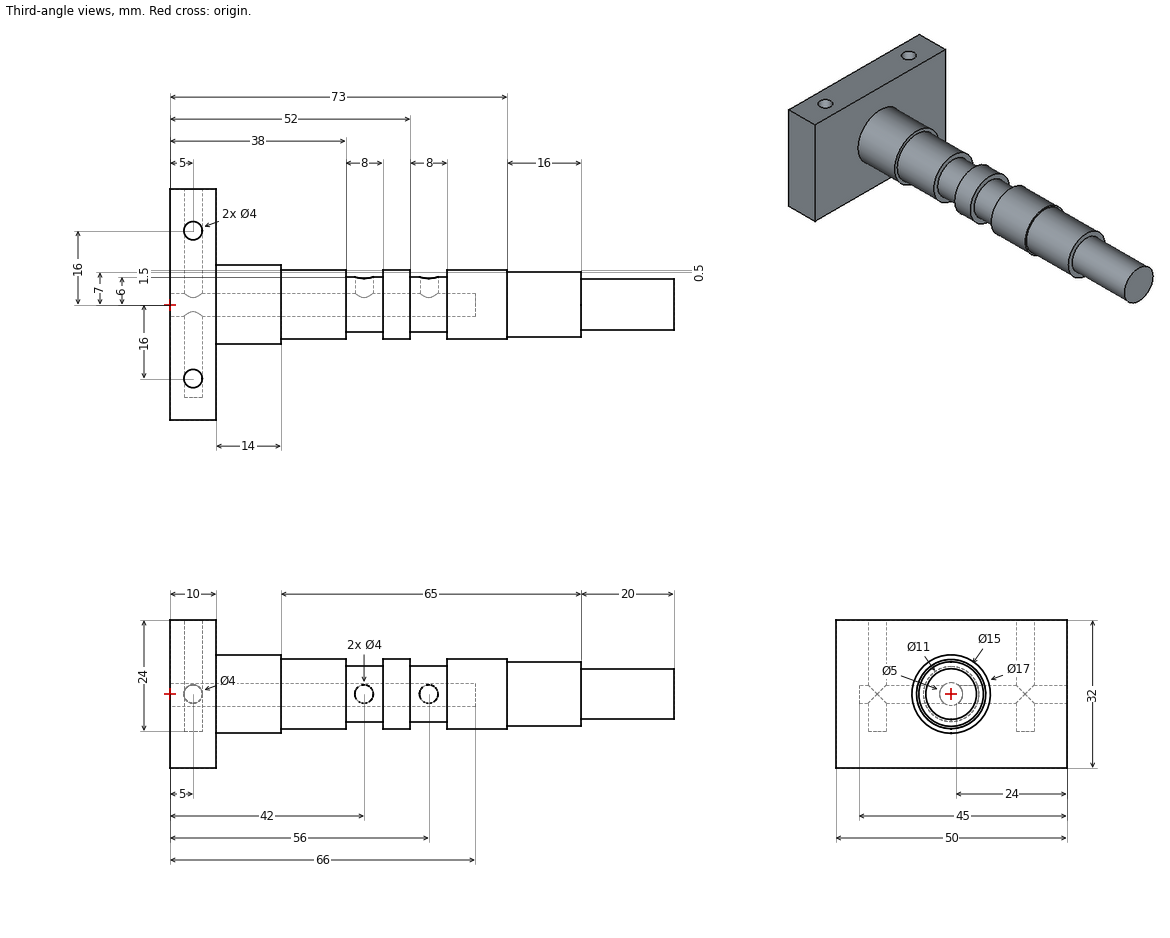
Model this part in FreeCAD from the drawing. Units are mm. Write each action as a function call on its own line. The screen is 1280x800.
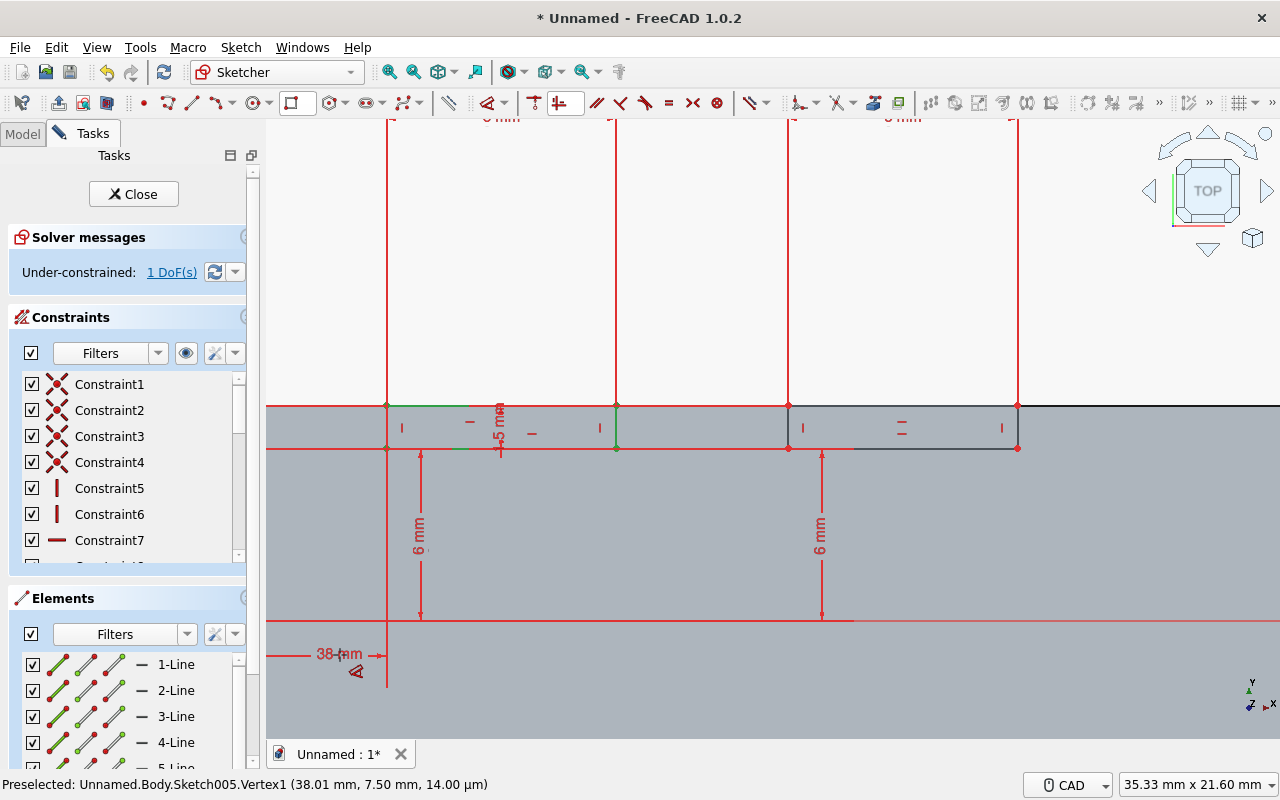
click(788, 406)
click(541, 655)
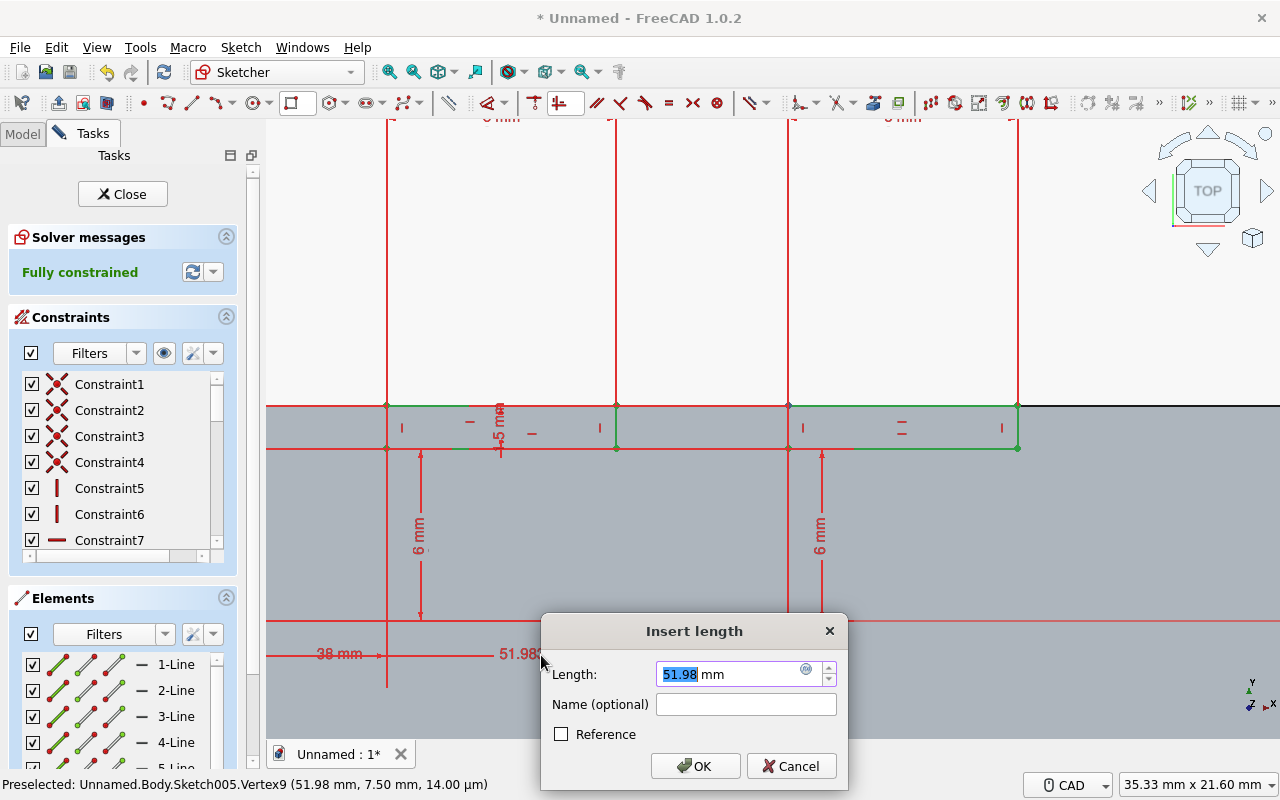
text(52)
key(Return)
key(Escape)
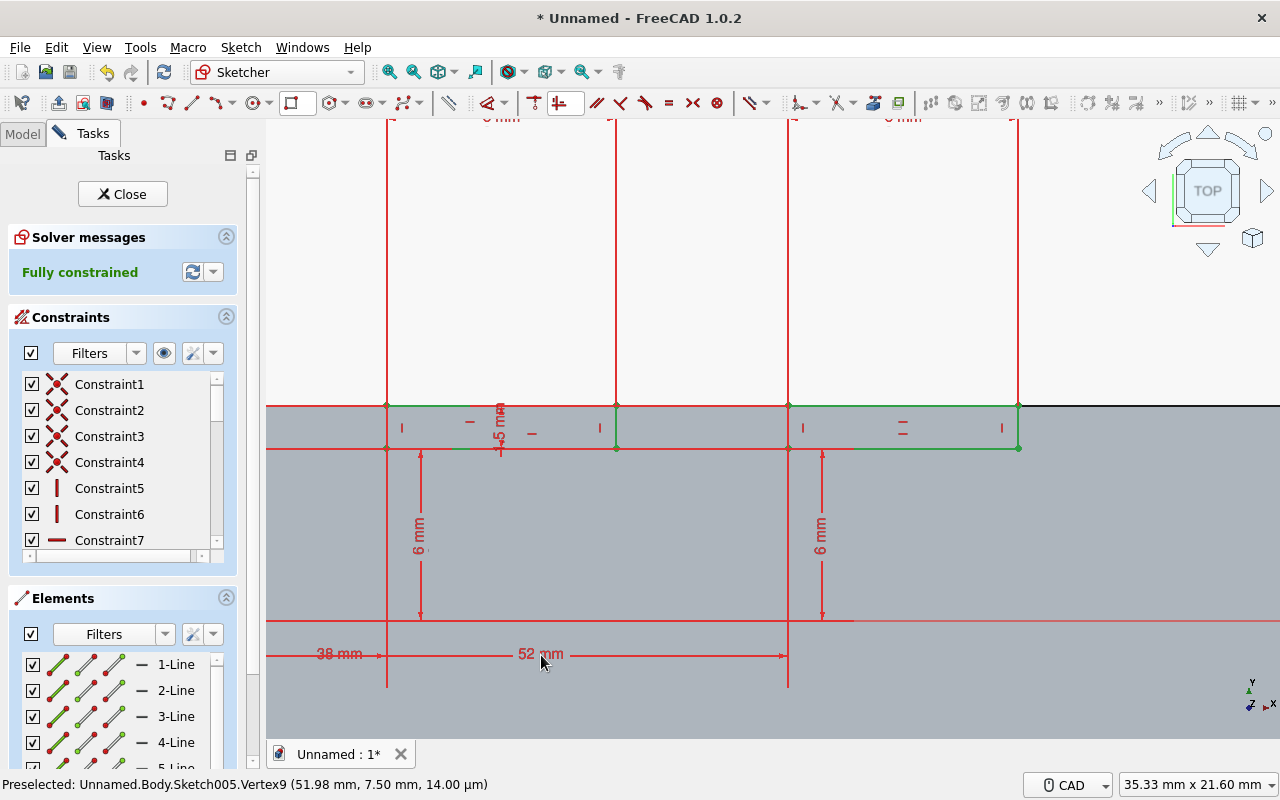
click(123, 194)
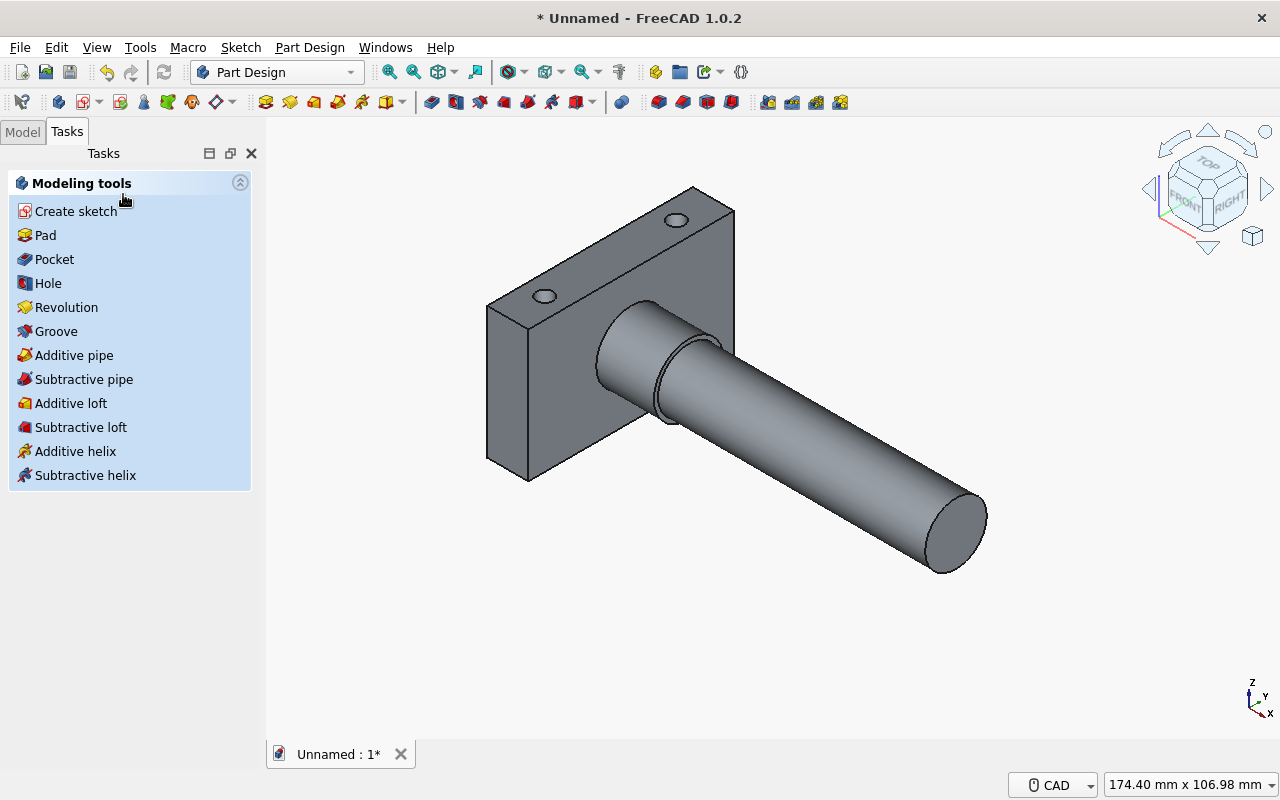
click(480, 102)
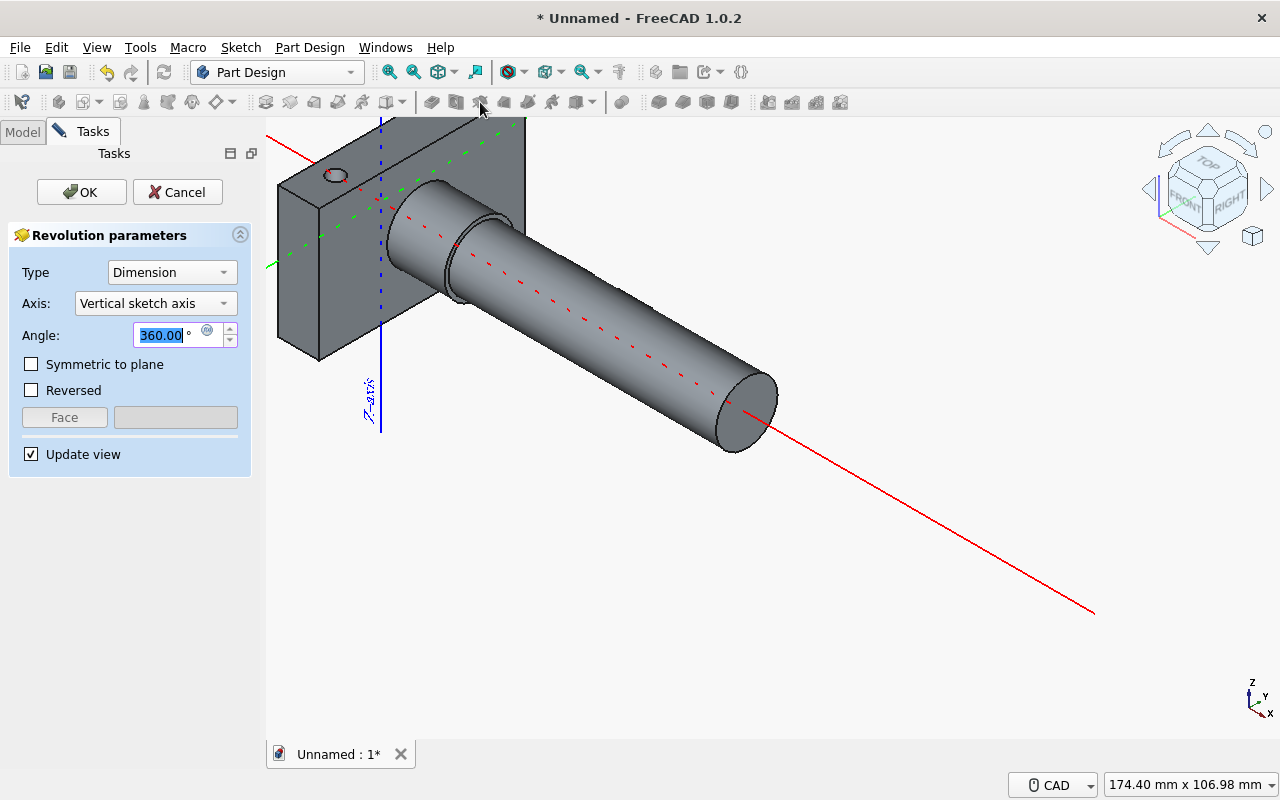
click(156, 304)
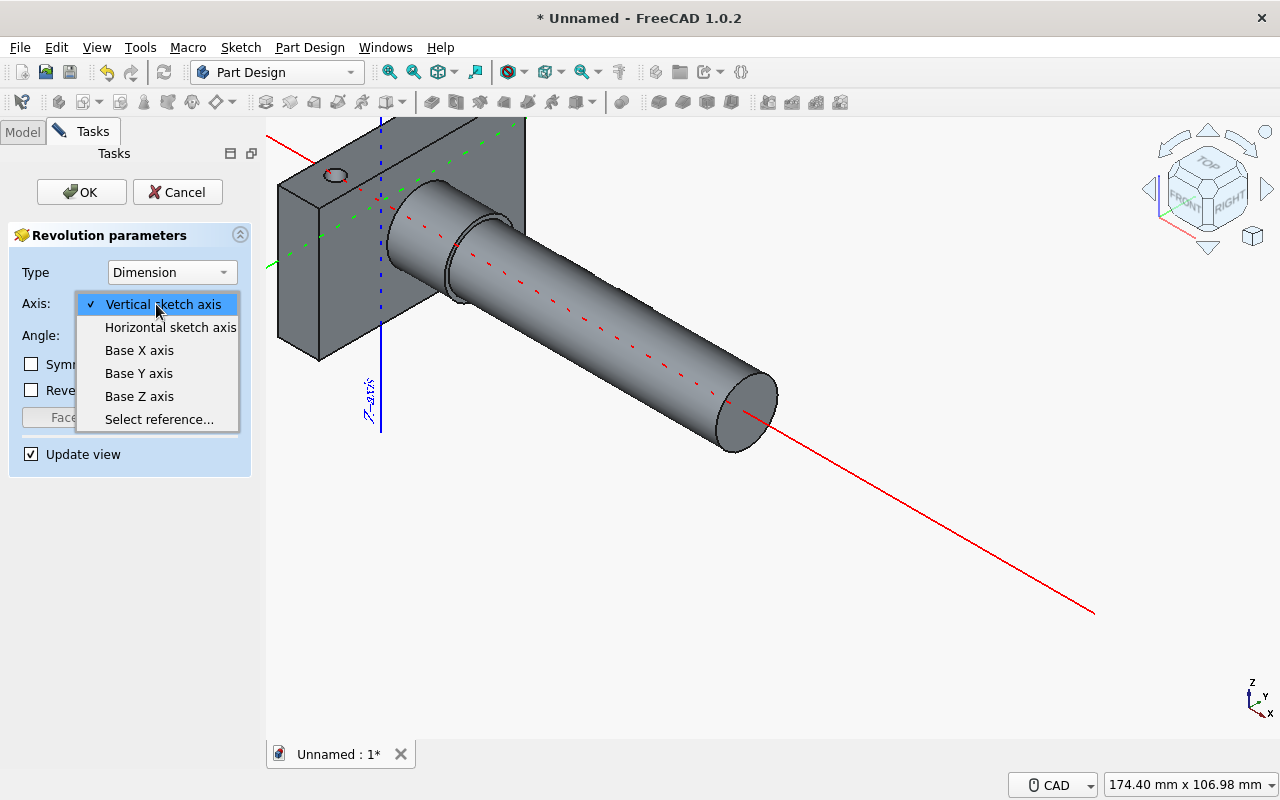
click(156, 328)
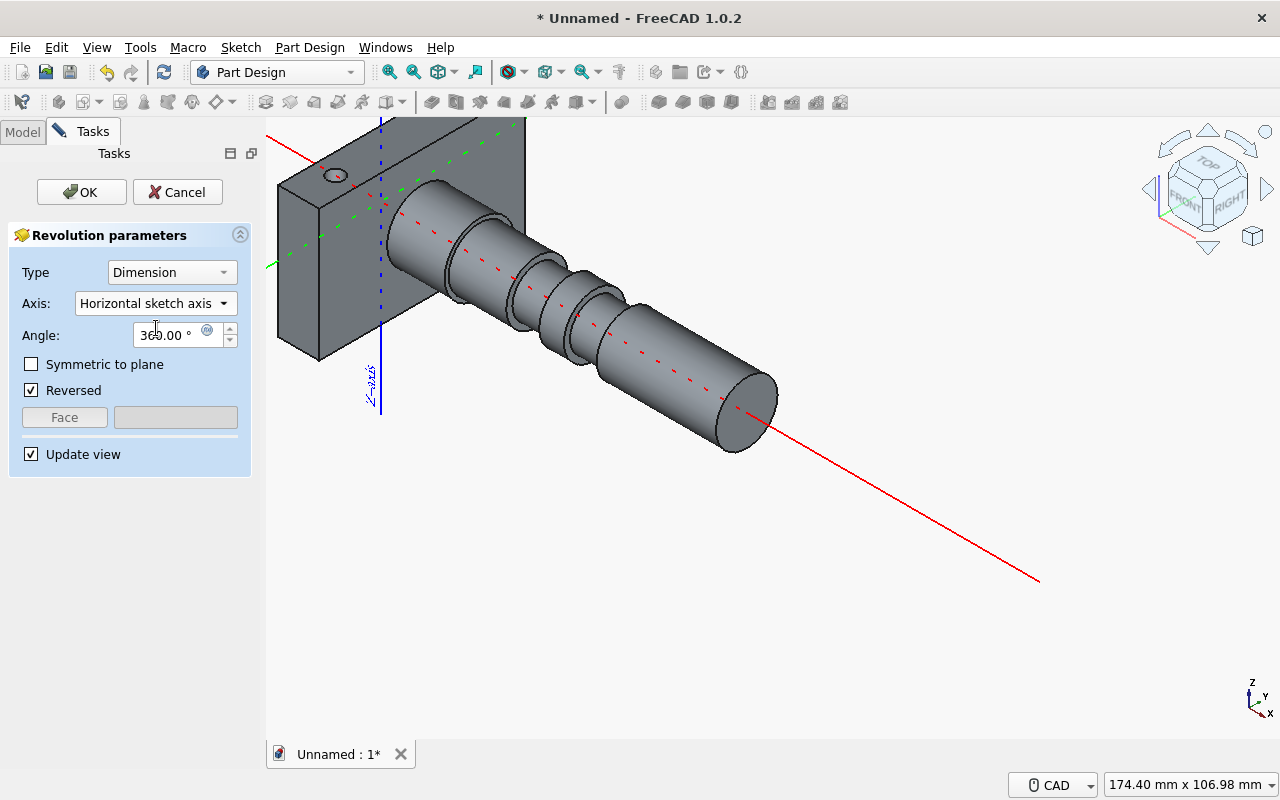
click(82, 192)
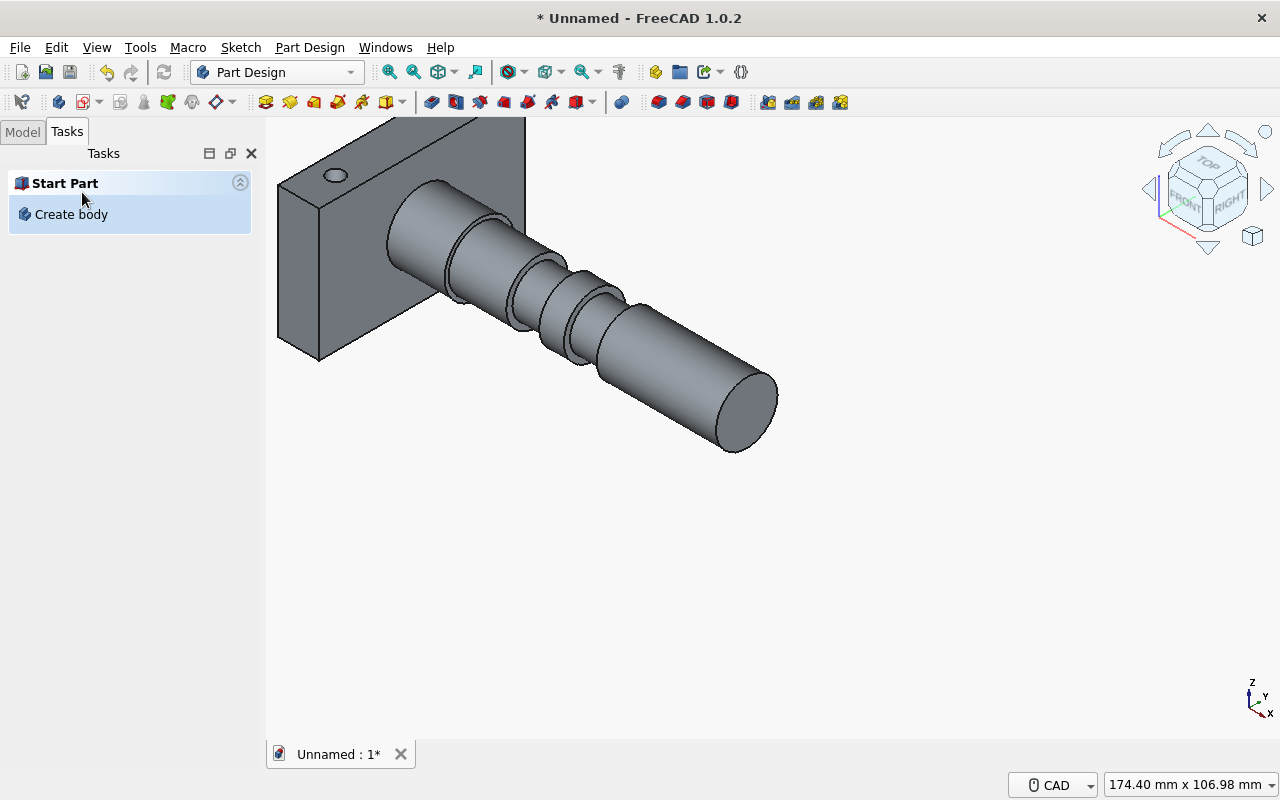
click(390, 72)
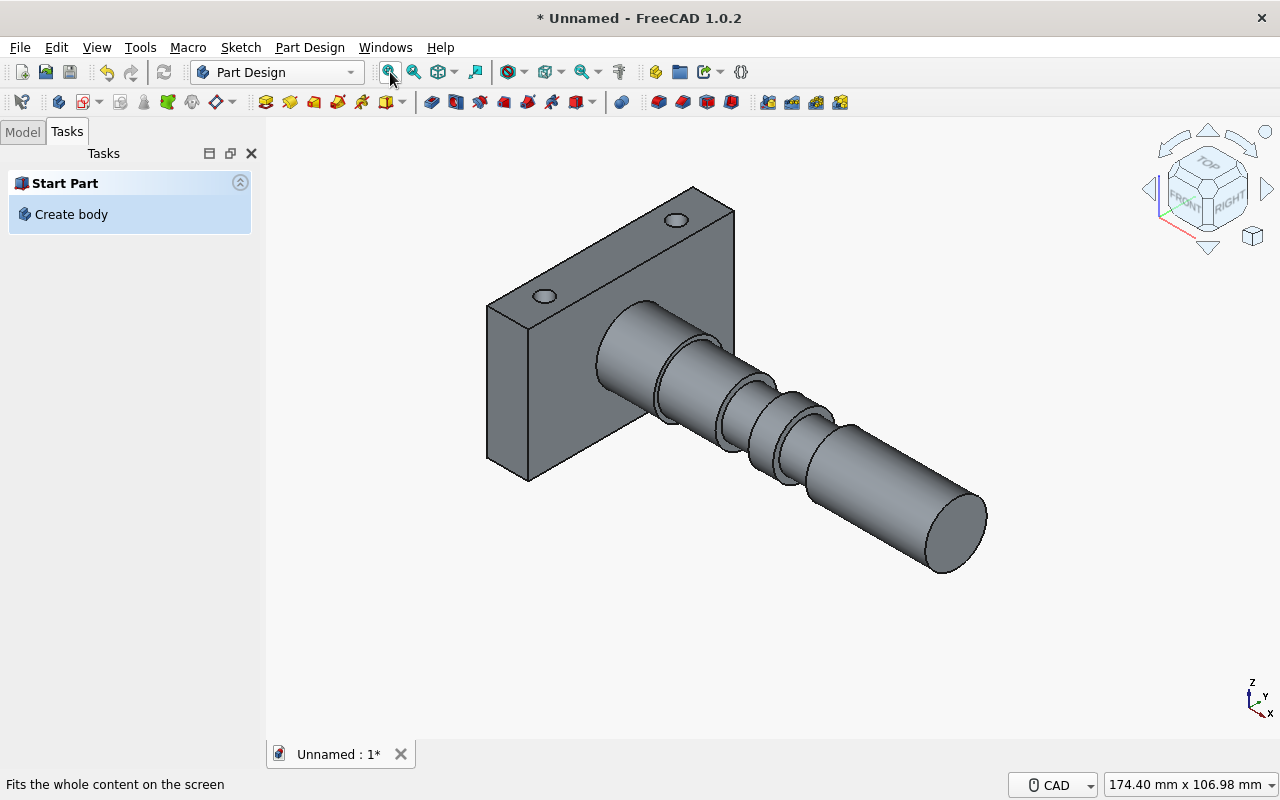
click(956, 533)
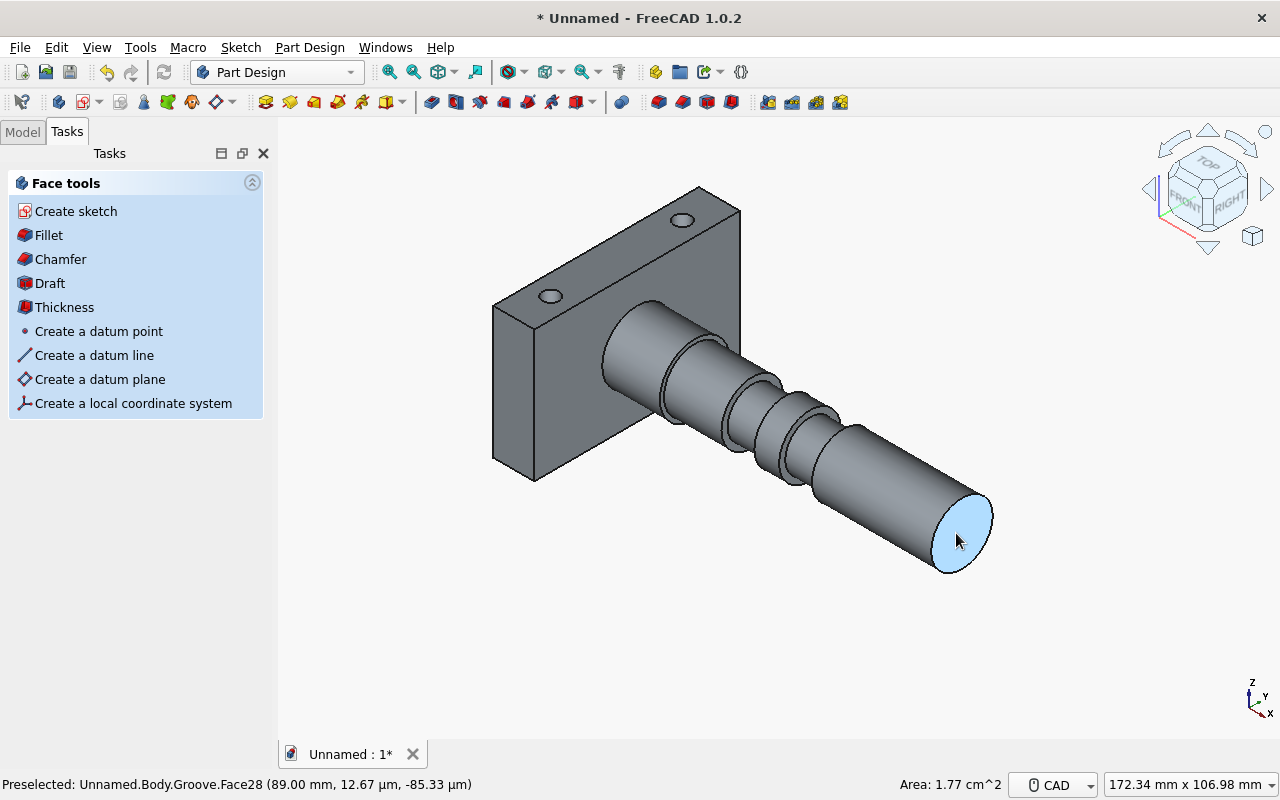
click(84, 102)